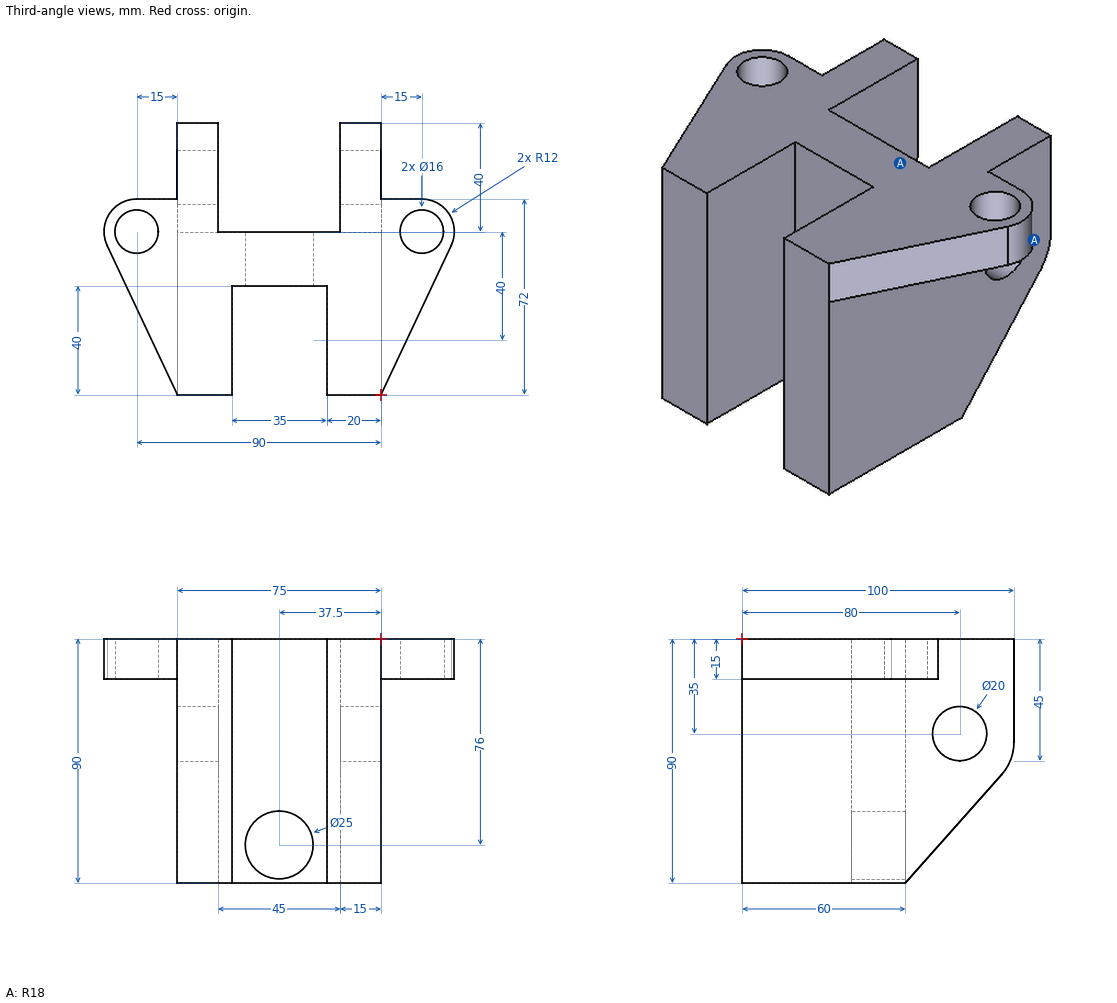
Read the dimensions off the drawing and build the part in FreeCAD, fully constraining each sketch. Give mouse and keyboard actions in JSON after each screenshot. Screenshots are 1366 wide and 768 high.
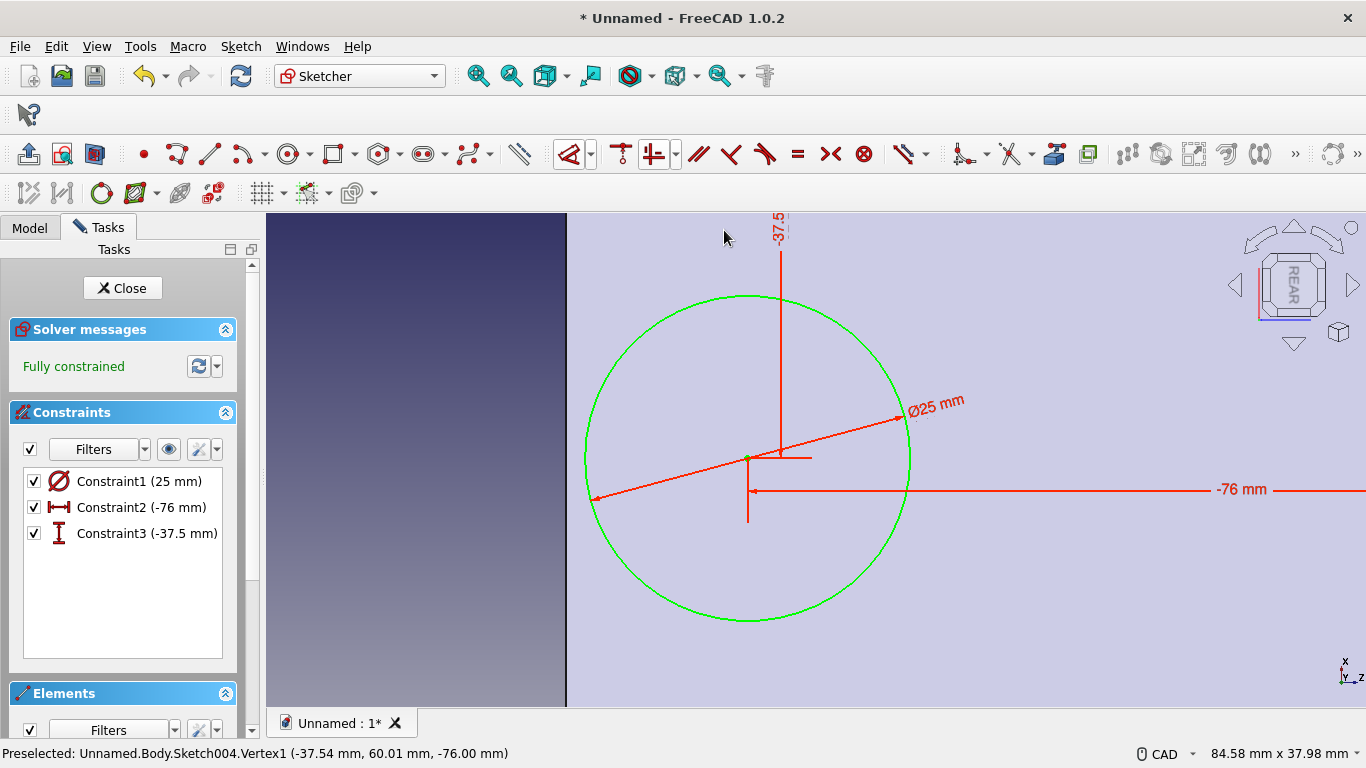
{"action": "left_click", "coordinate": [123, 288]}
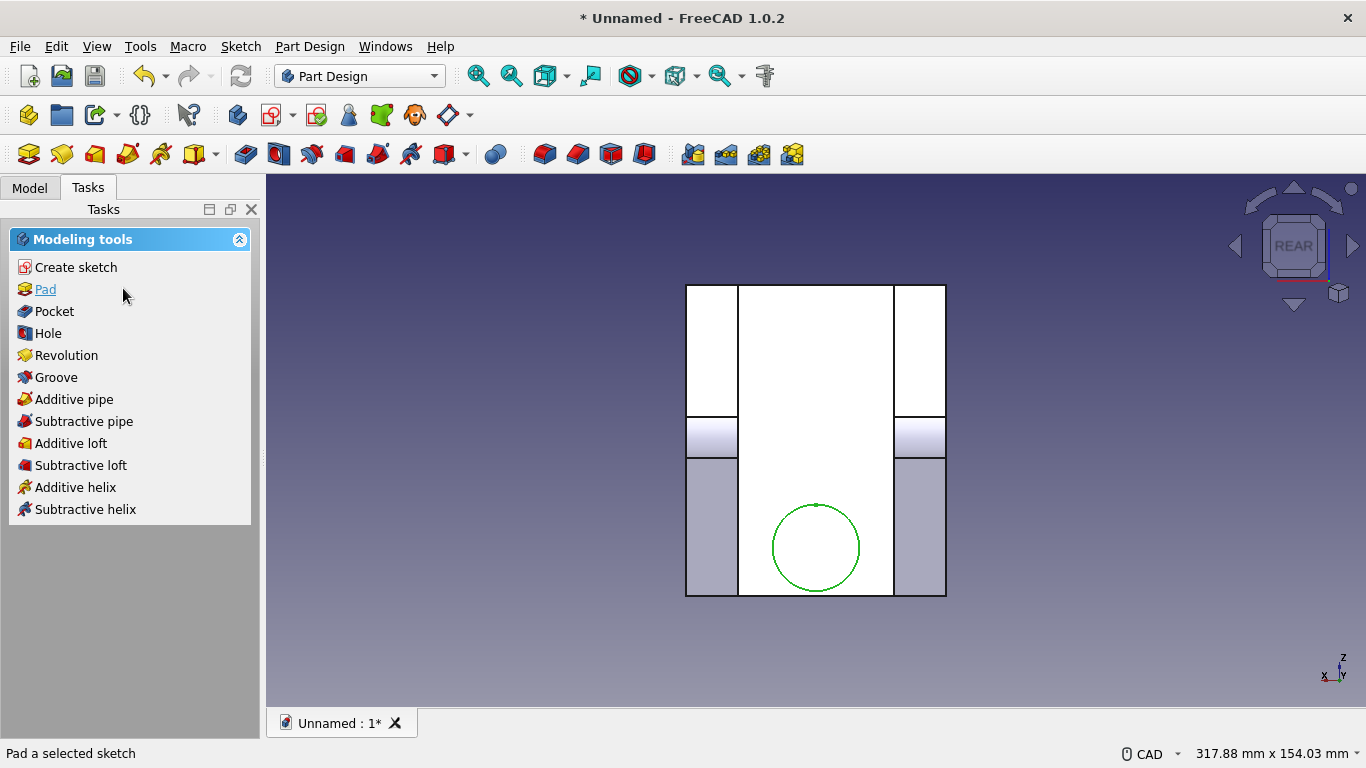
{"action": "left_click", "coordinate": [246, 154]}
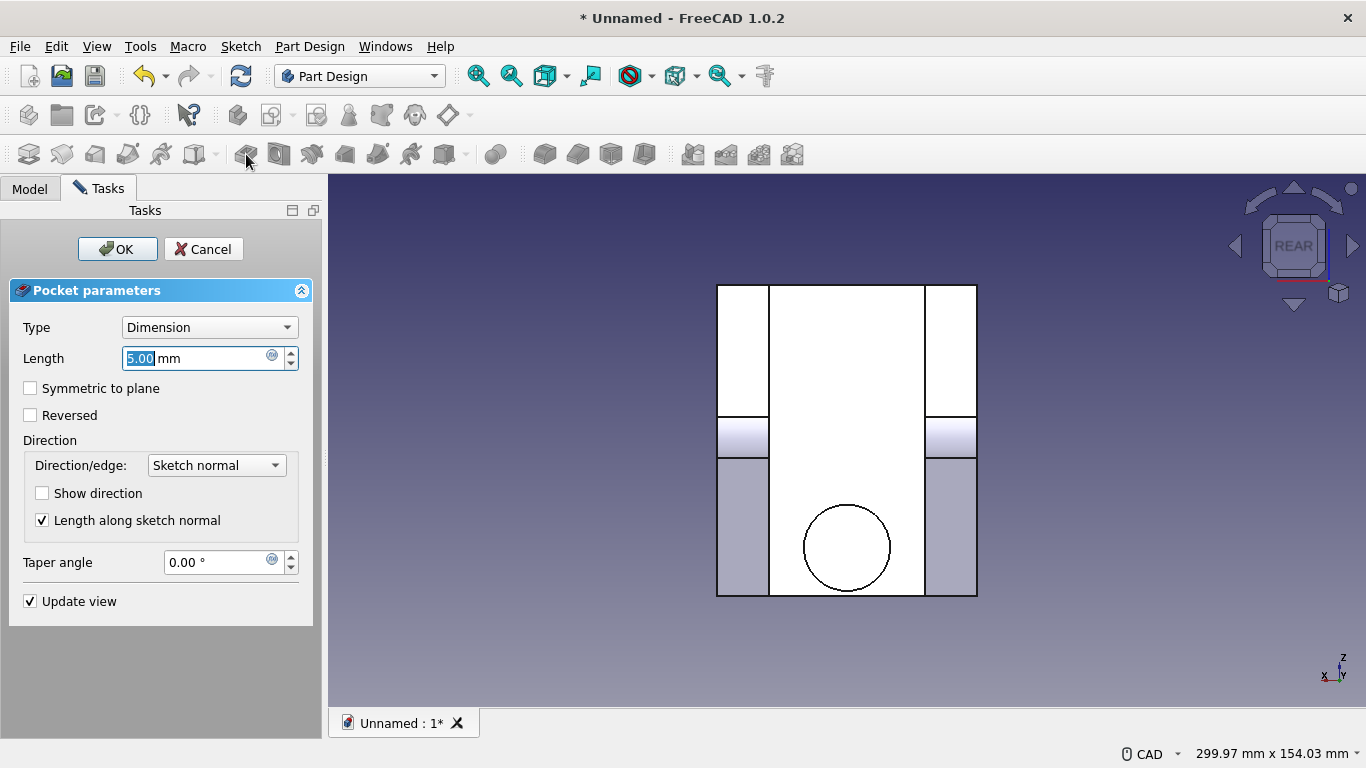
{"action": "type", "text": "40"}
{"action": "key", "text": "Tab"}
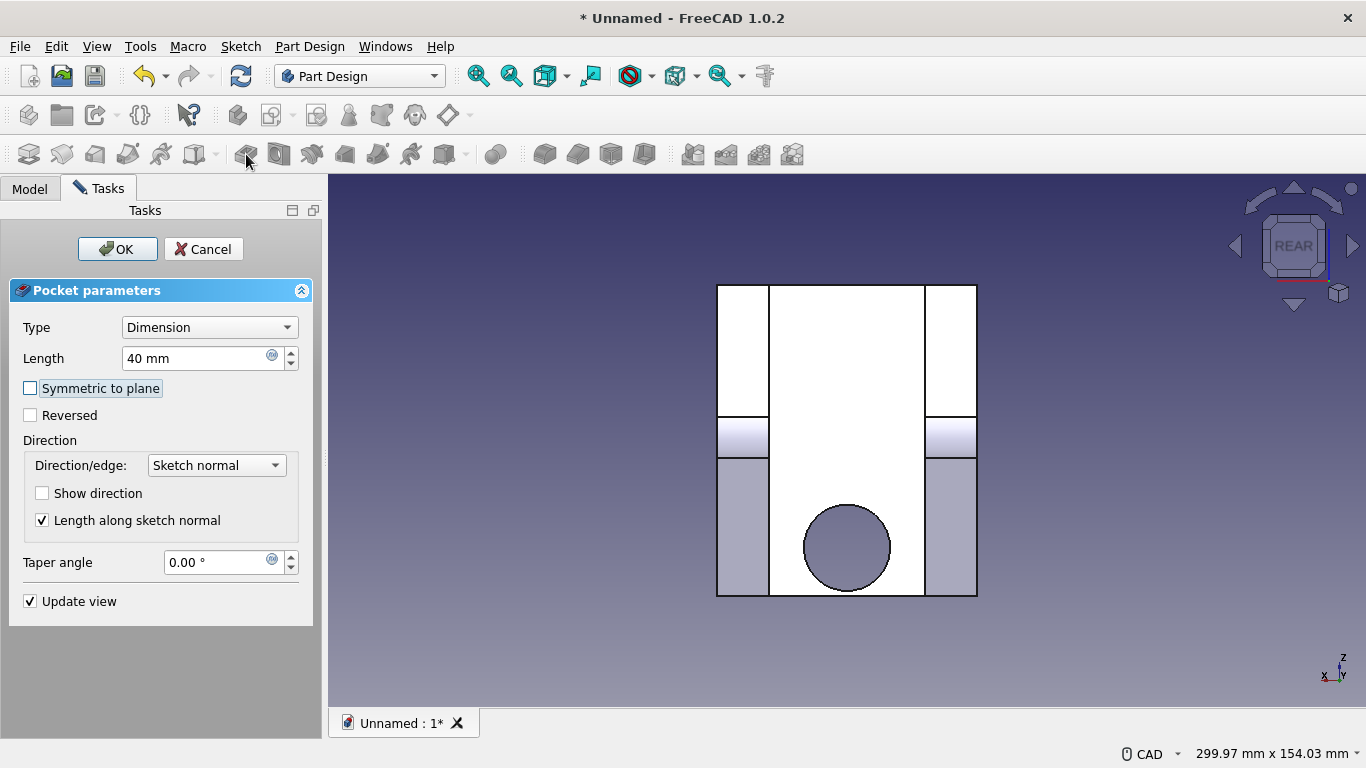
{"action": "left_click", "coordinate": [118, 249]}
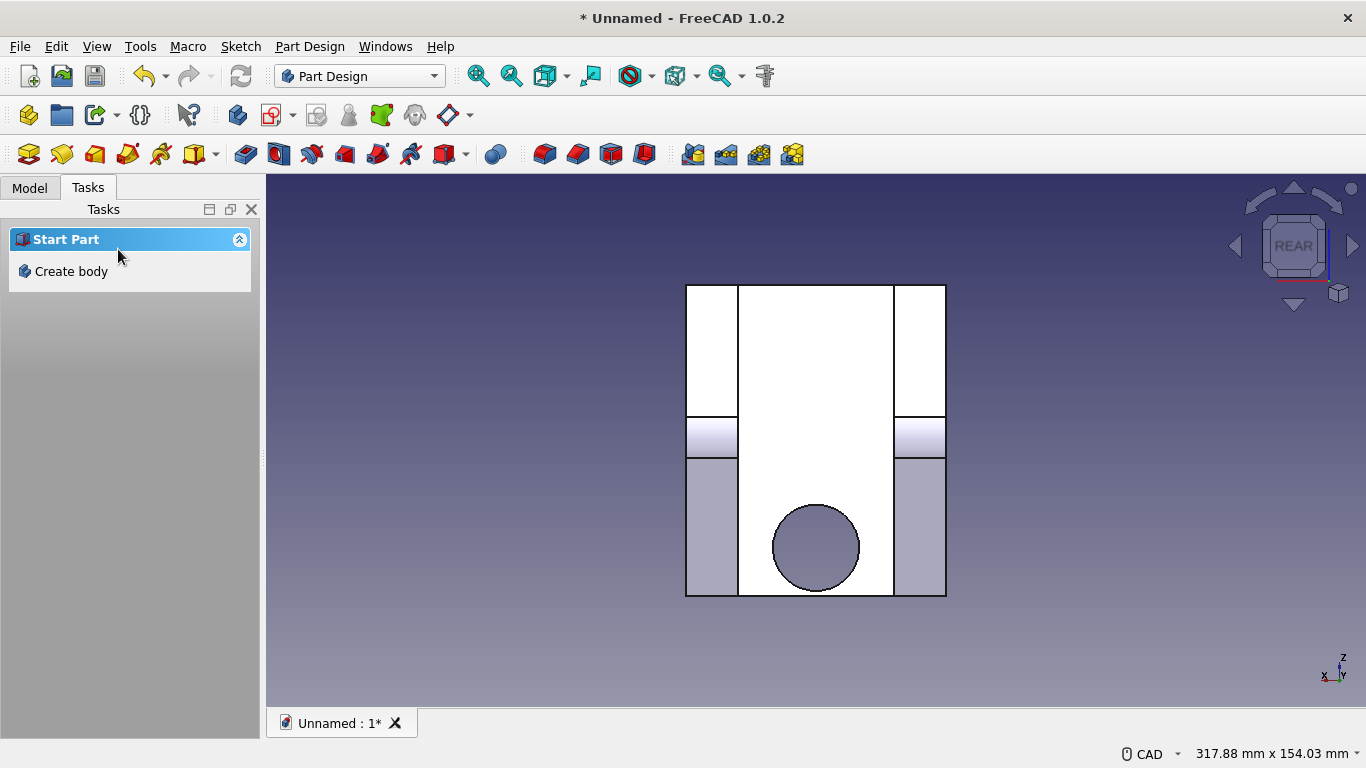
{"action": "key", "text": "0"}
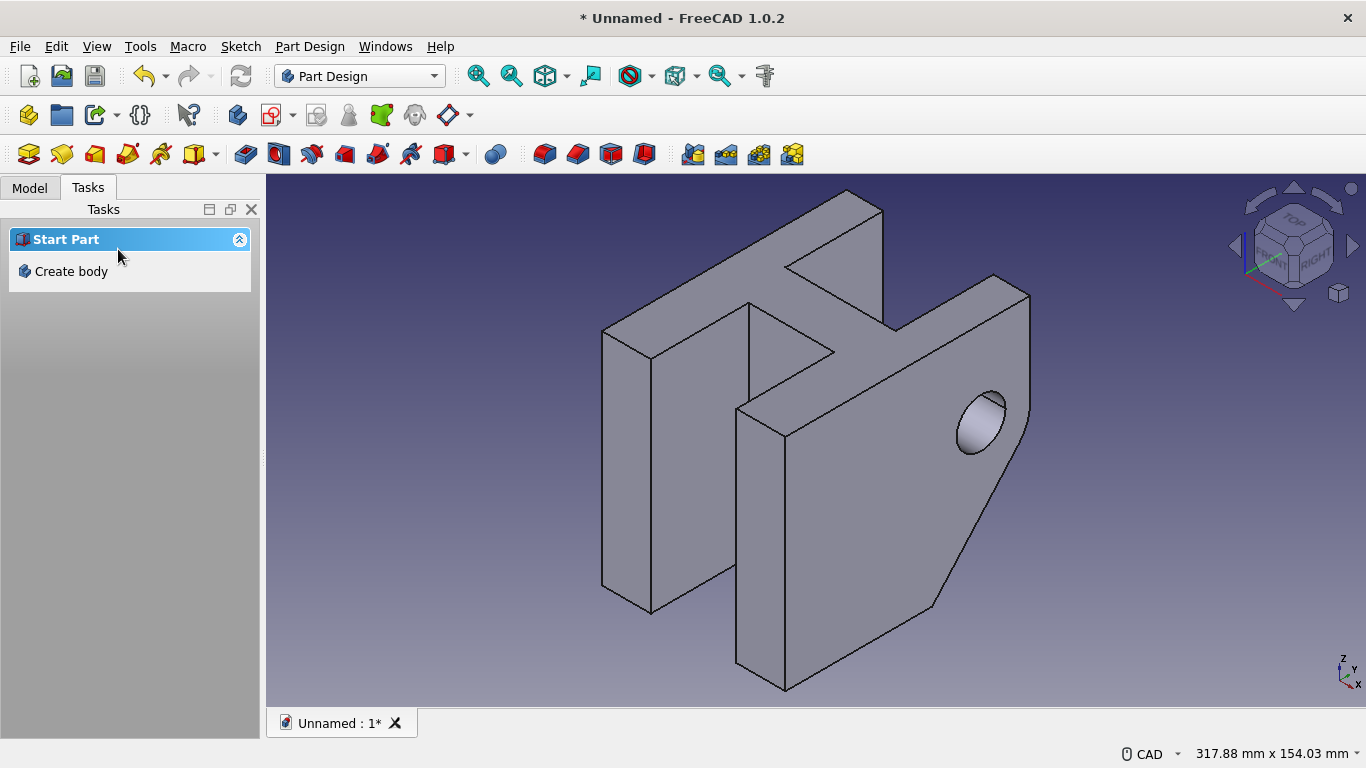
{"action": "left_click", "coordinate": [868, 343]}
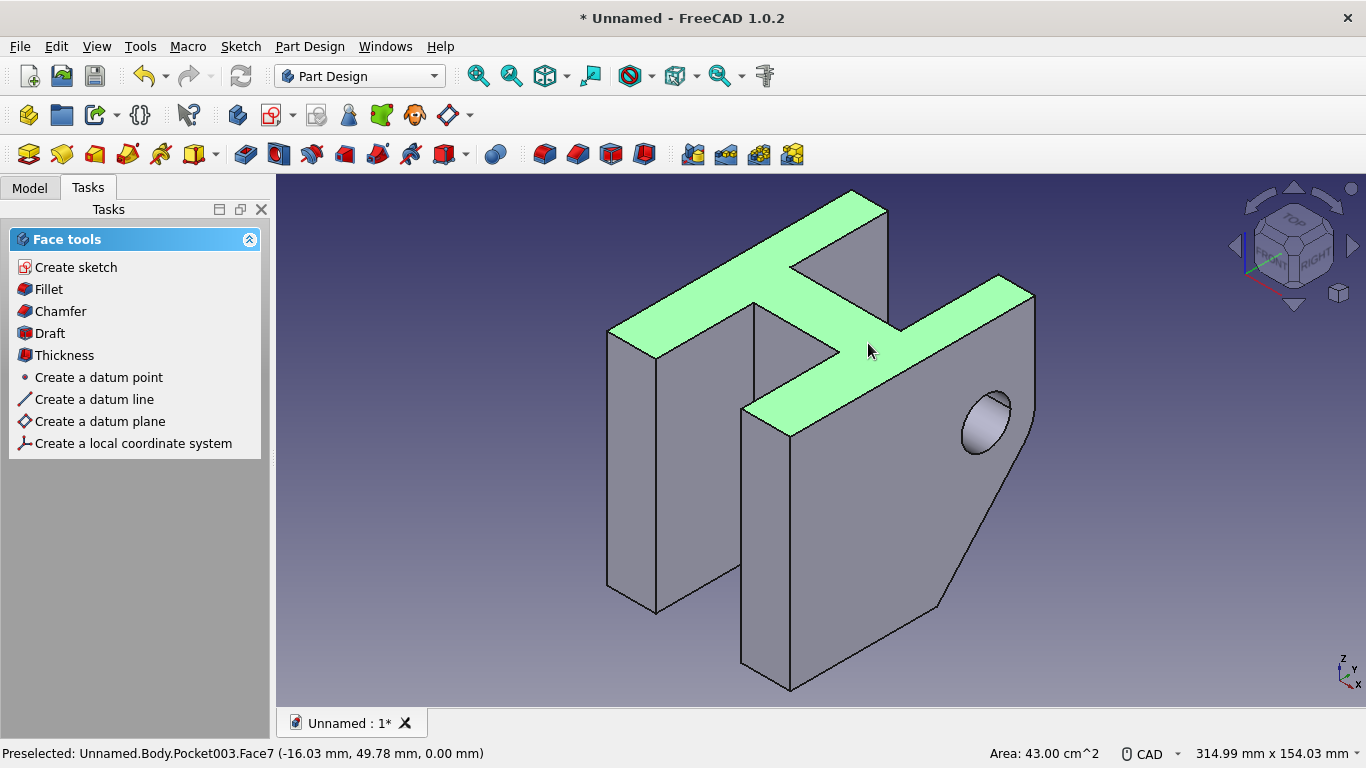
{"action": "left_click", "coordinate": [270, 116]}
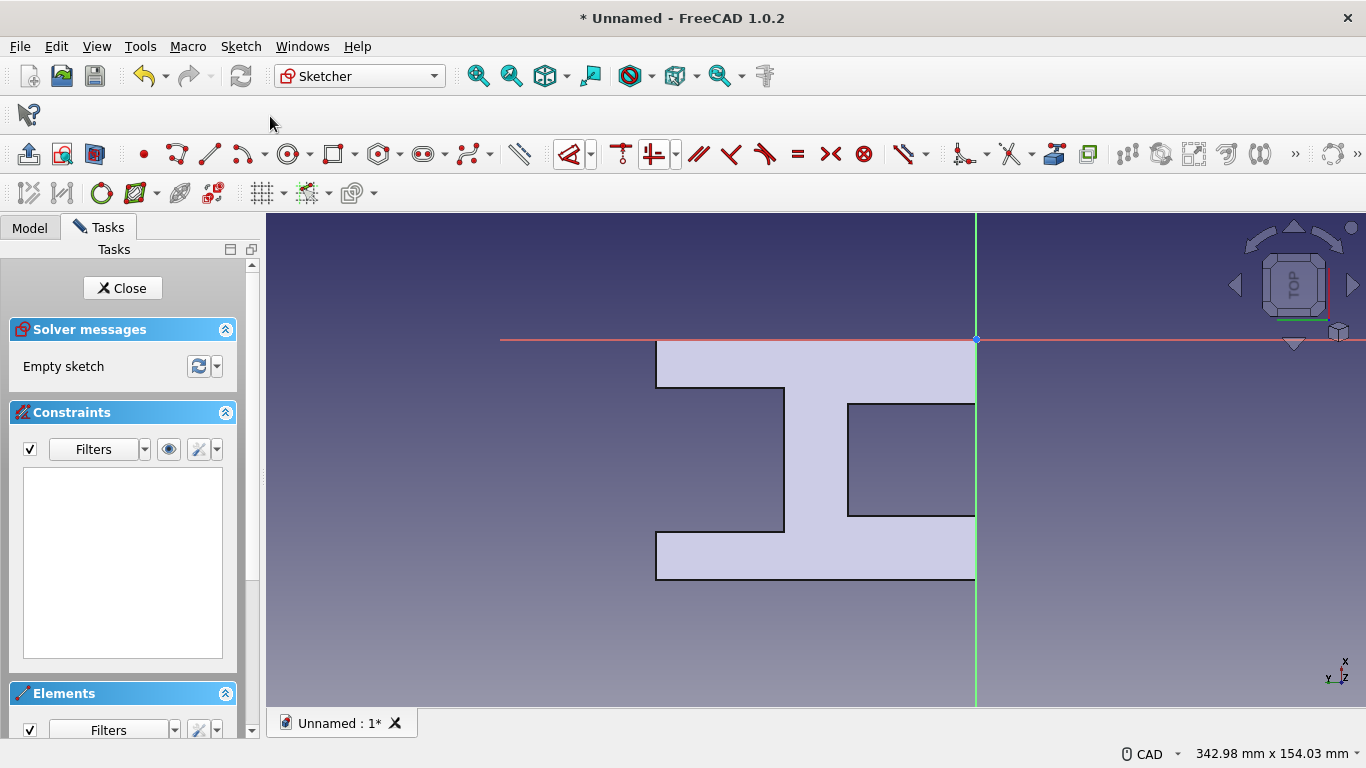
{"action": "scroll", "coordinate": [294, 460], "scroll_direction": "down", "scroll_amount": 1}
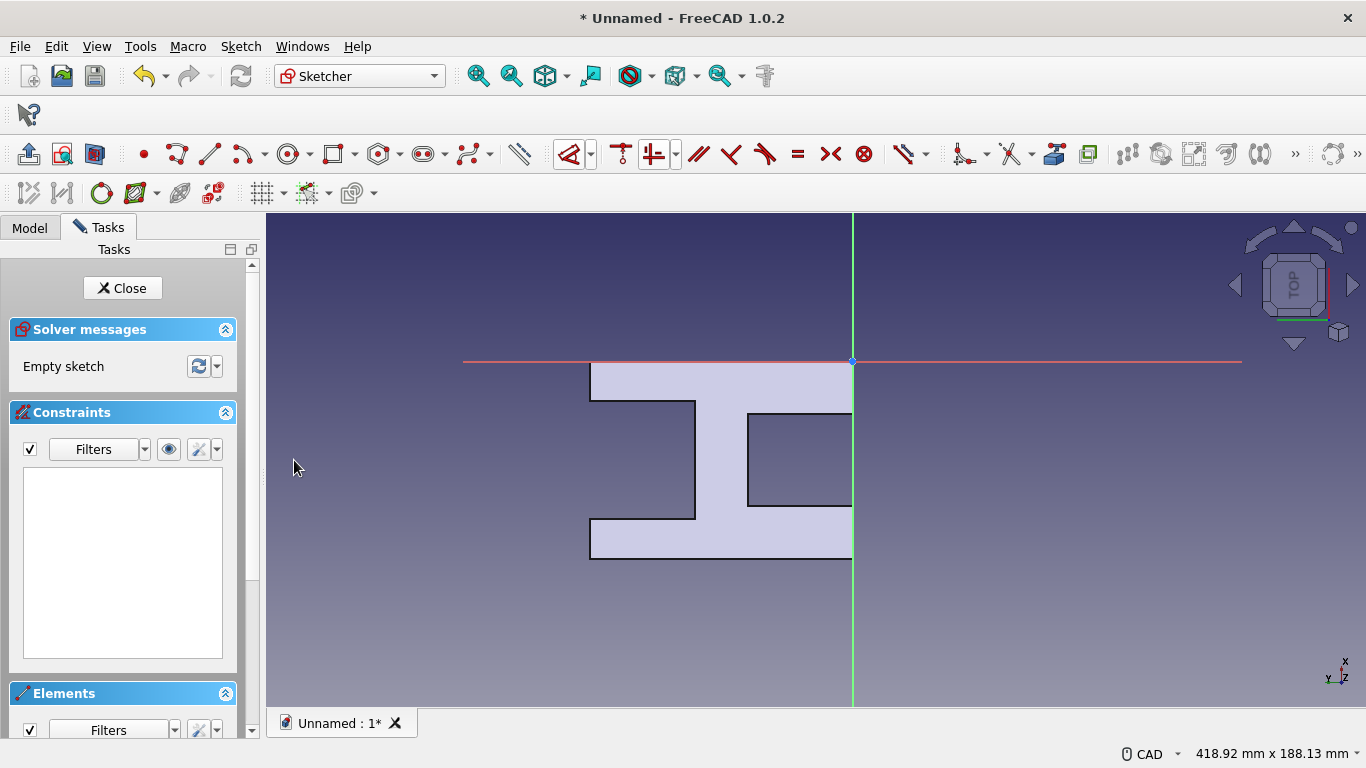
{"action": "key", "text": "g m"}